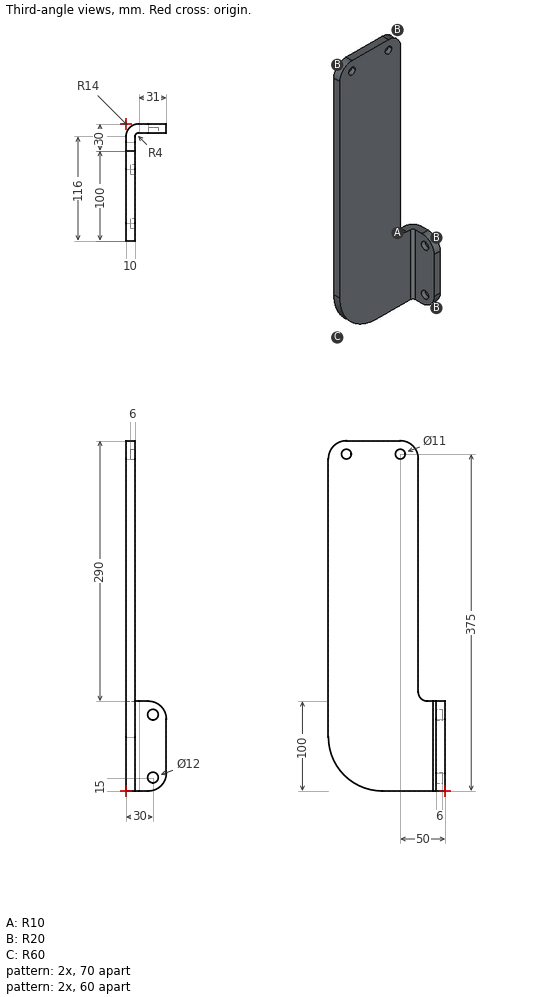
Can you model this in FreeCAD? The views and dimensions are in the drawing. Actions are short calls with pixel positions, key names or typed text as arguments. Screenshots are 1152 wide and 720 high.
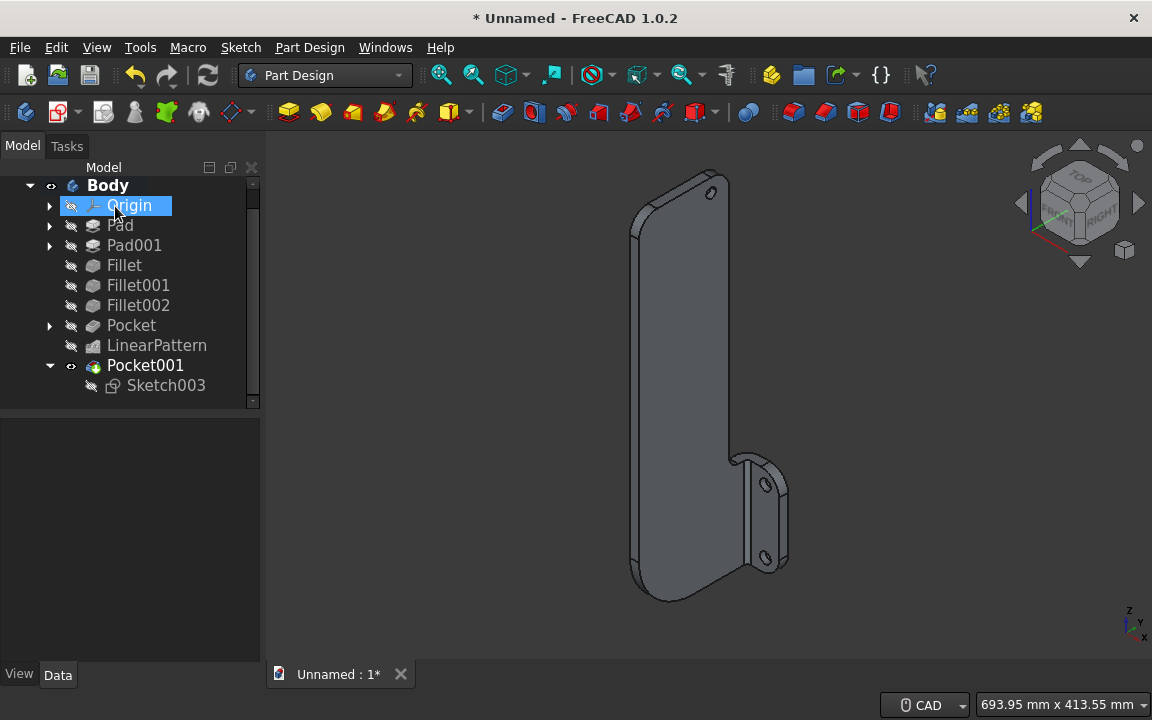
click(116, 366)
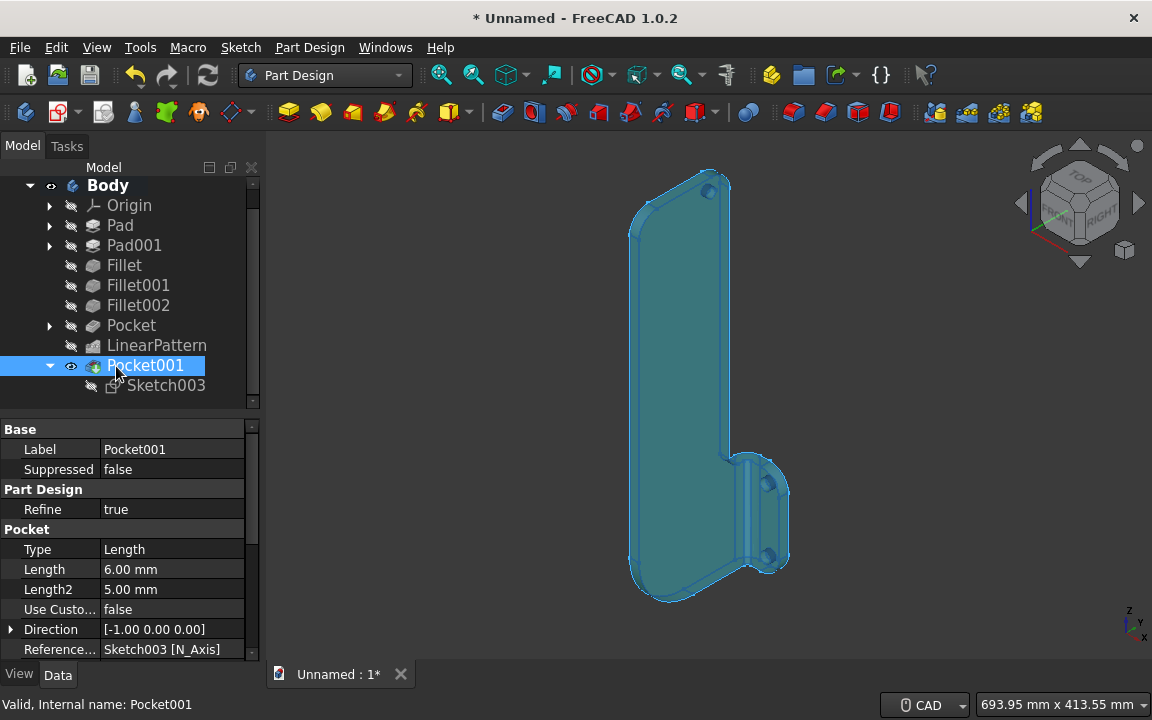
click(968, 112)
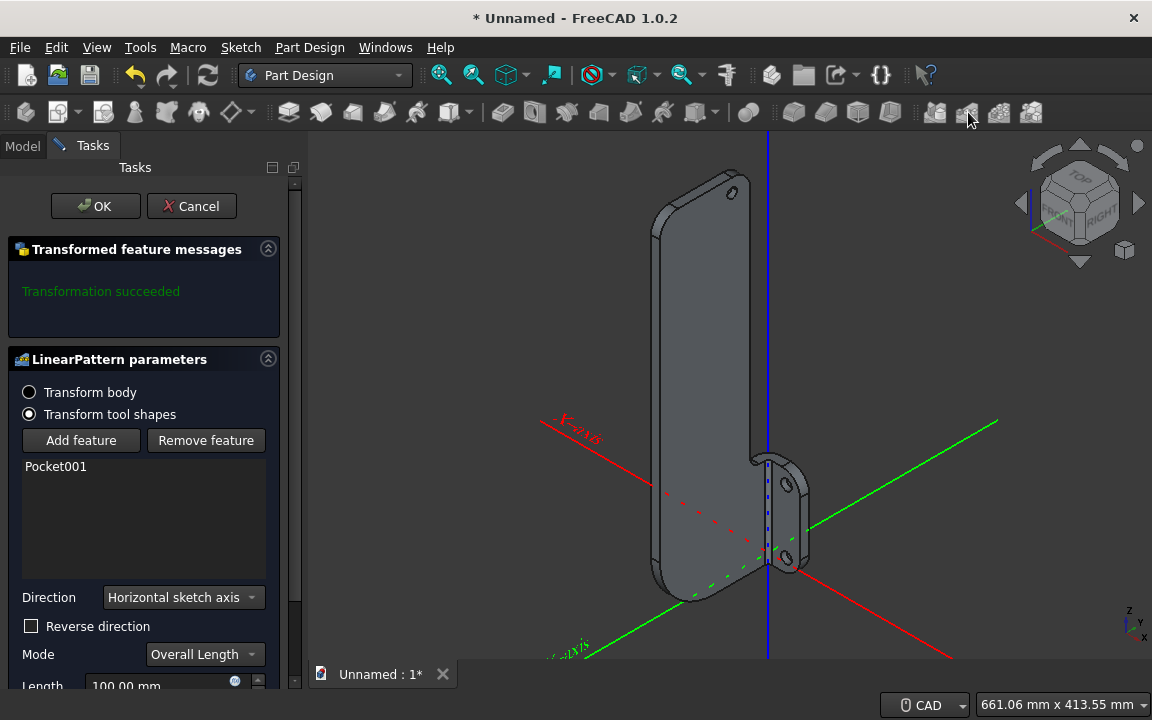
click(184, 598)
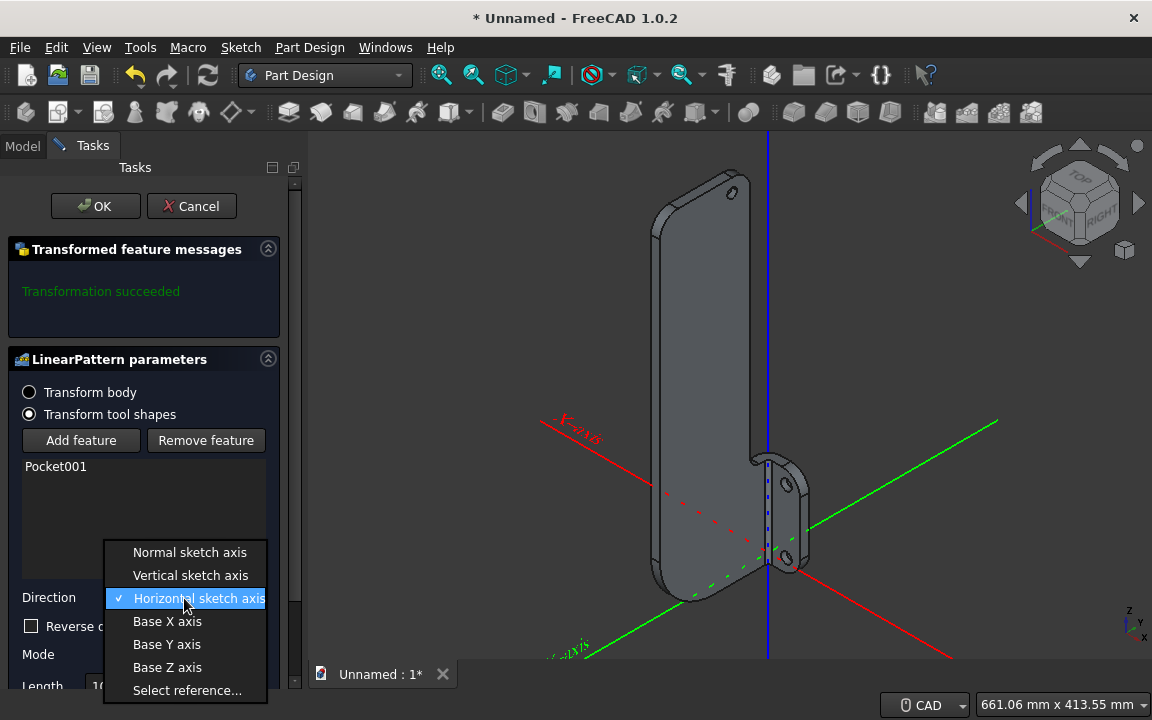
click(184, 644)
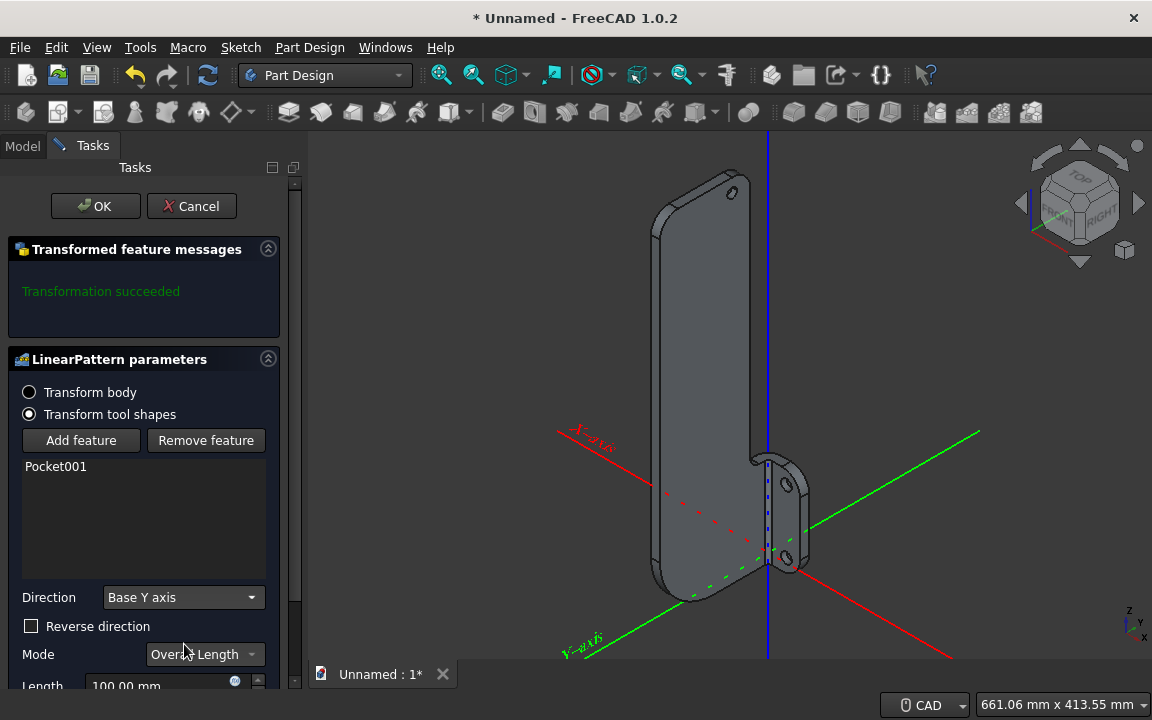
click(206, 654)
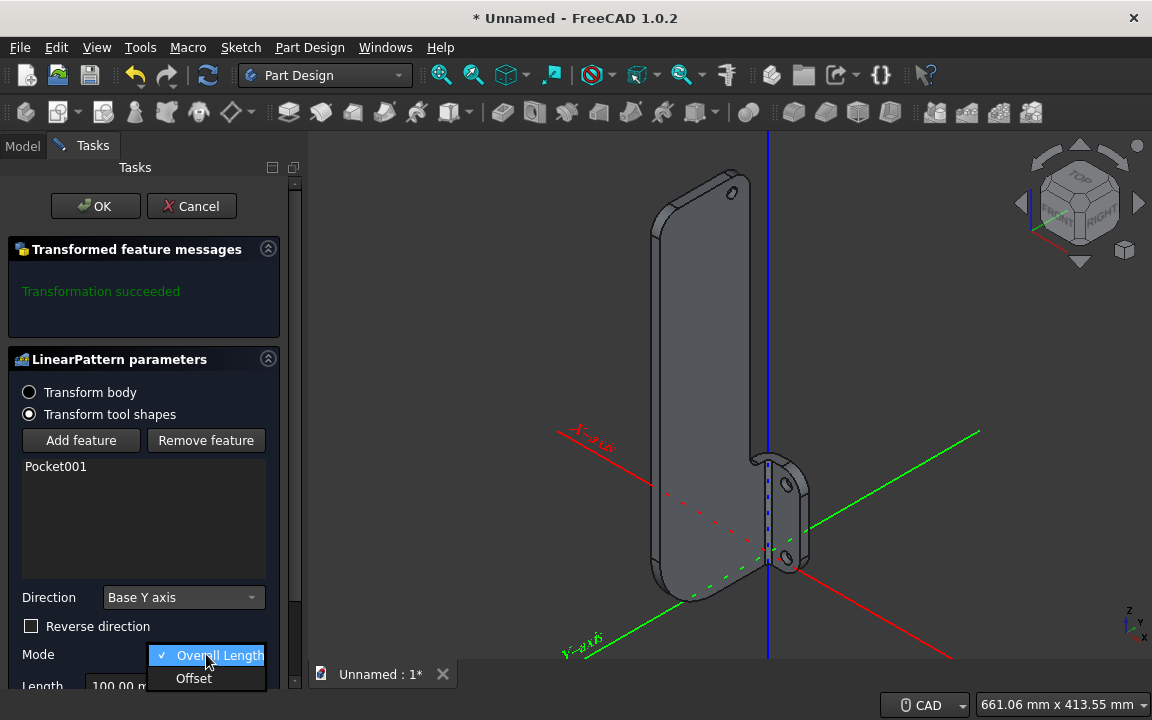
click(206, 678)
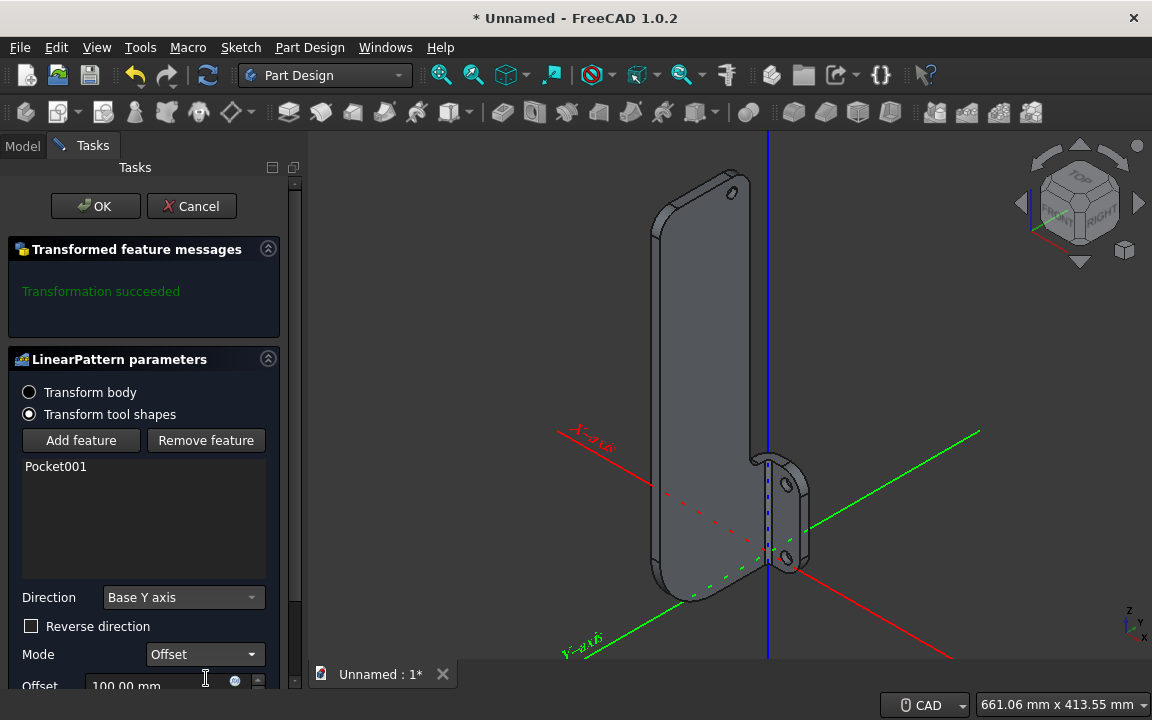
scroll(295, 432, down, 2)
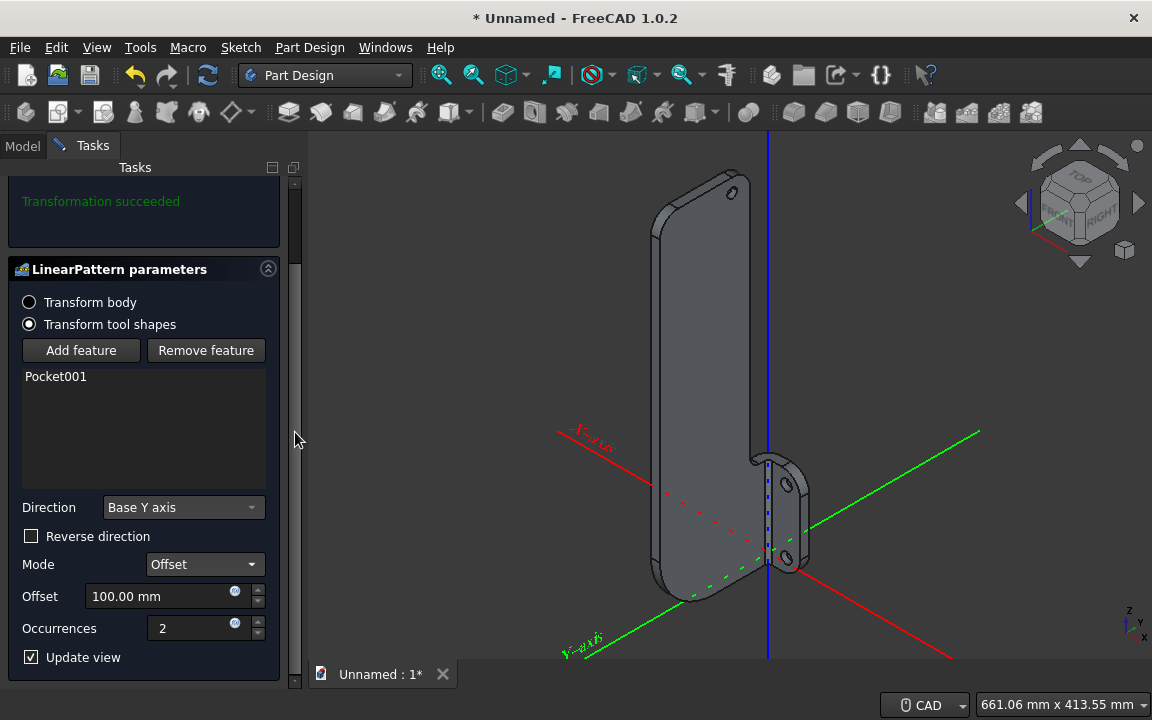
triple_click(168, 596)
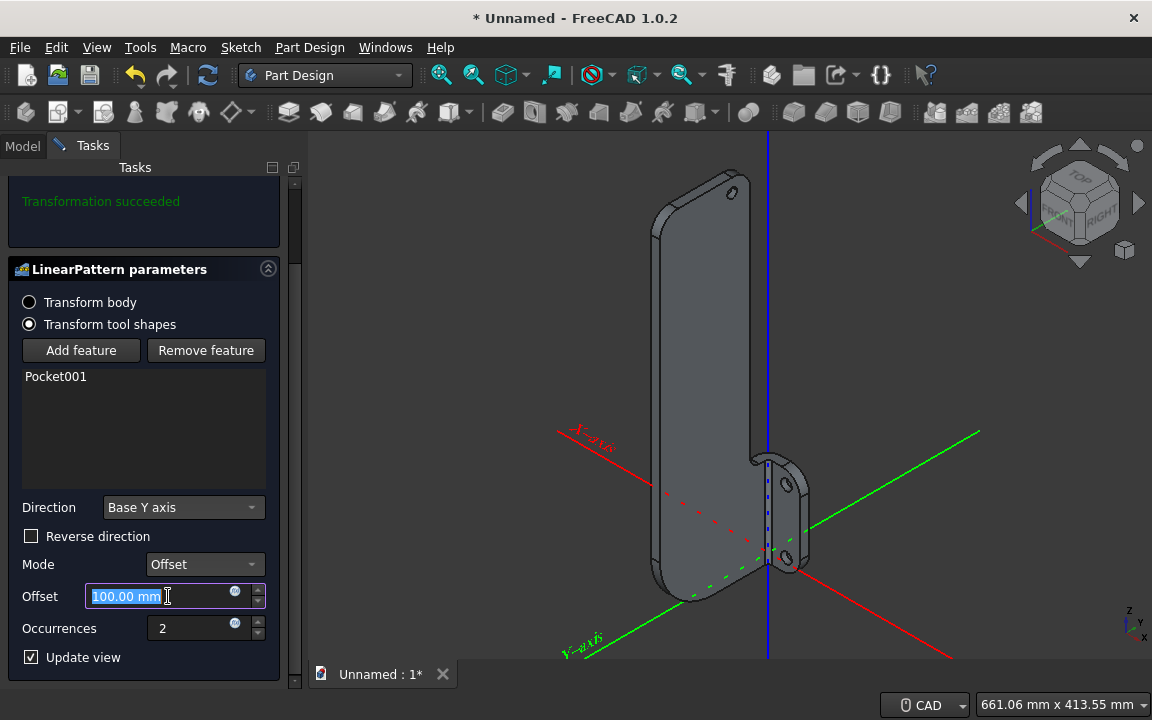
text(60)
key(Tab)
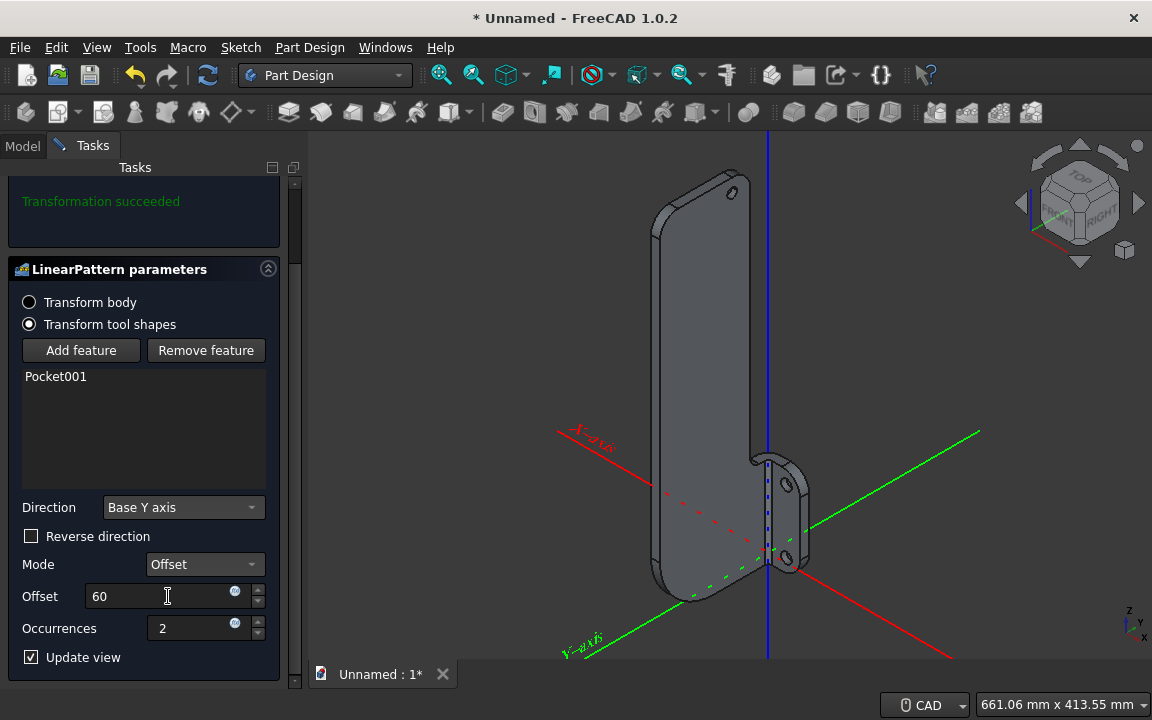
triple_click(198, 628)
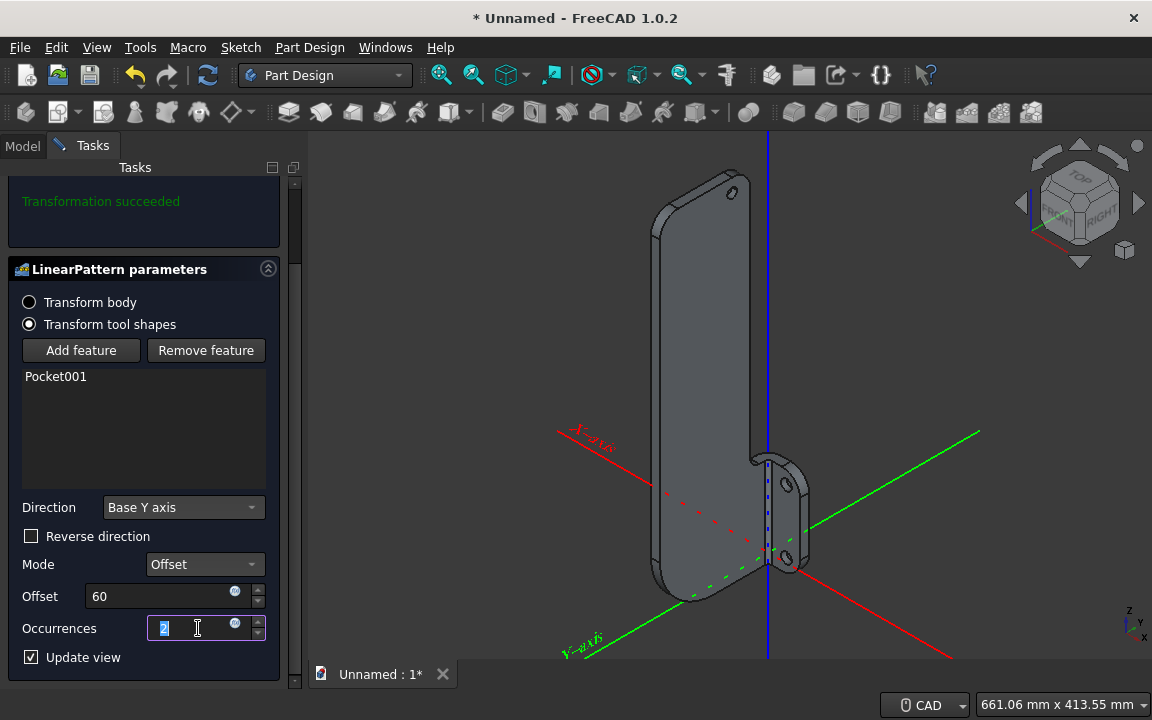
text(2)
key(Tab)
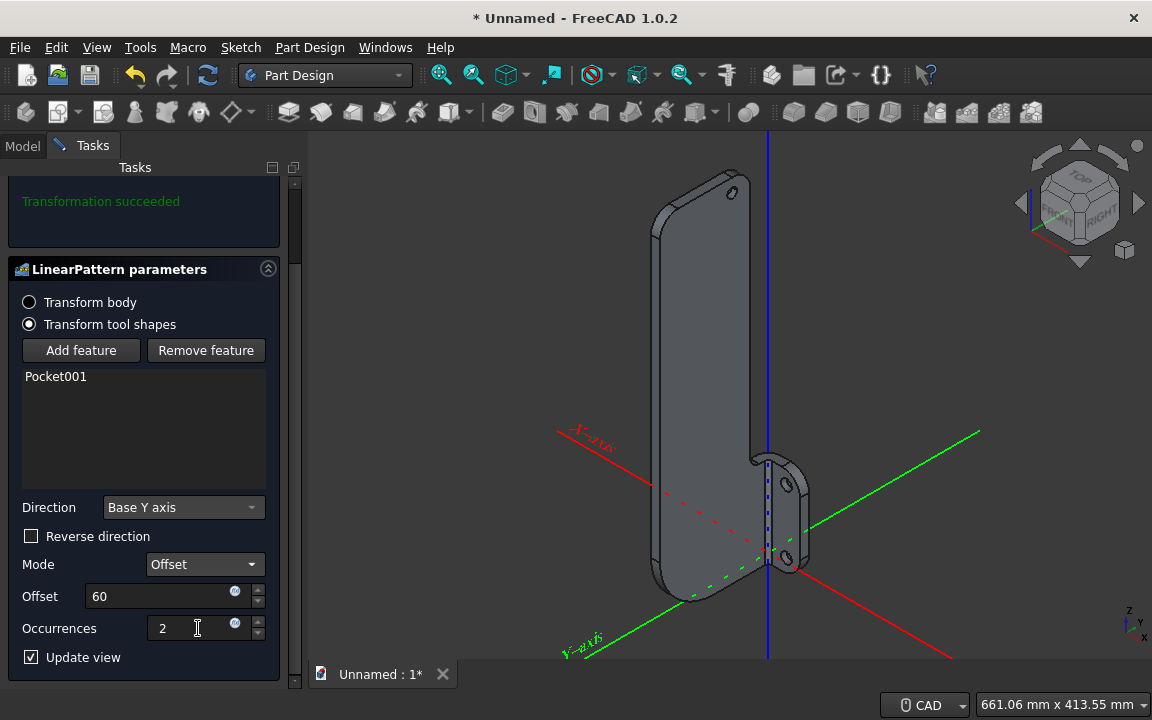
click(30, 536)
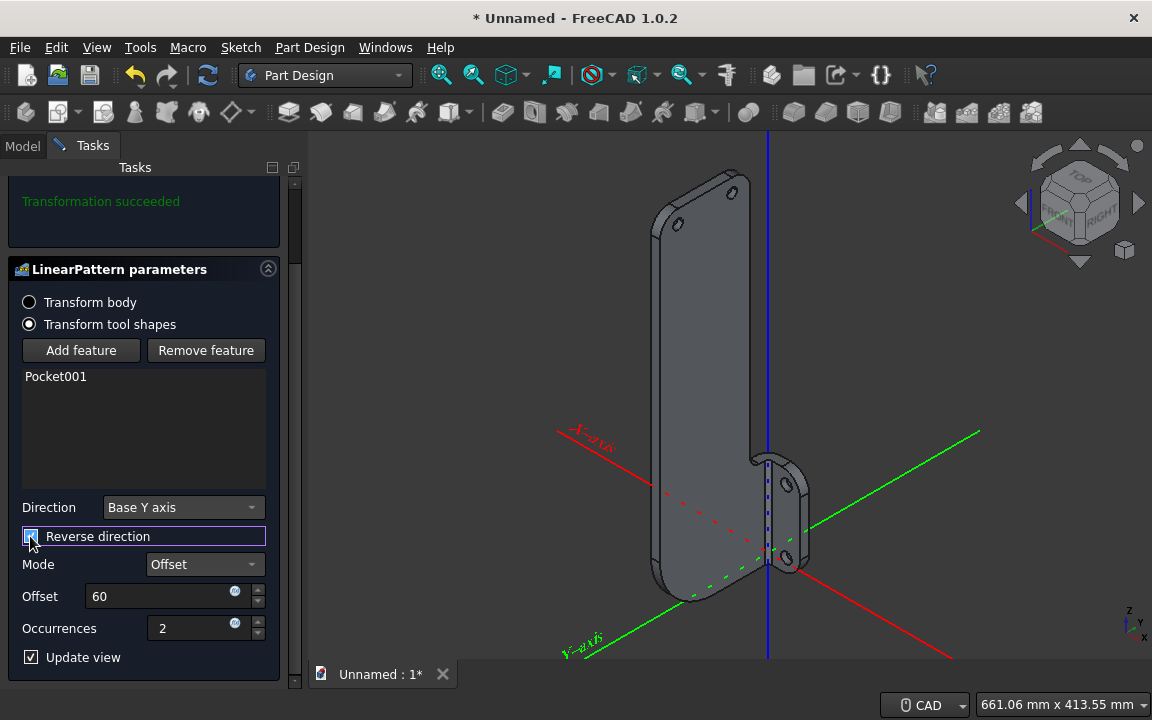
scroll(295, 432, up, 3)